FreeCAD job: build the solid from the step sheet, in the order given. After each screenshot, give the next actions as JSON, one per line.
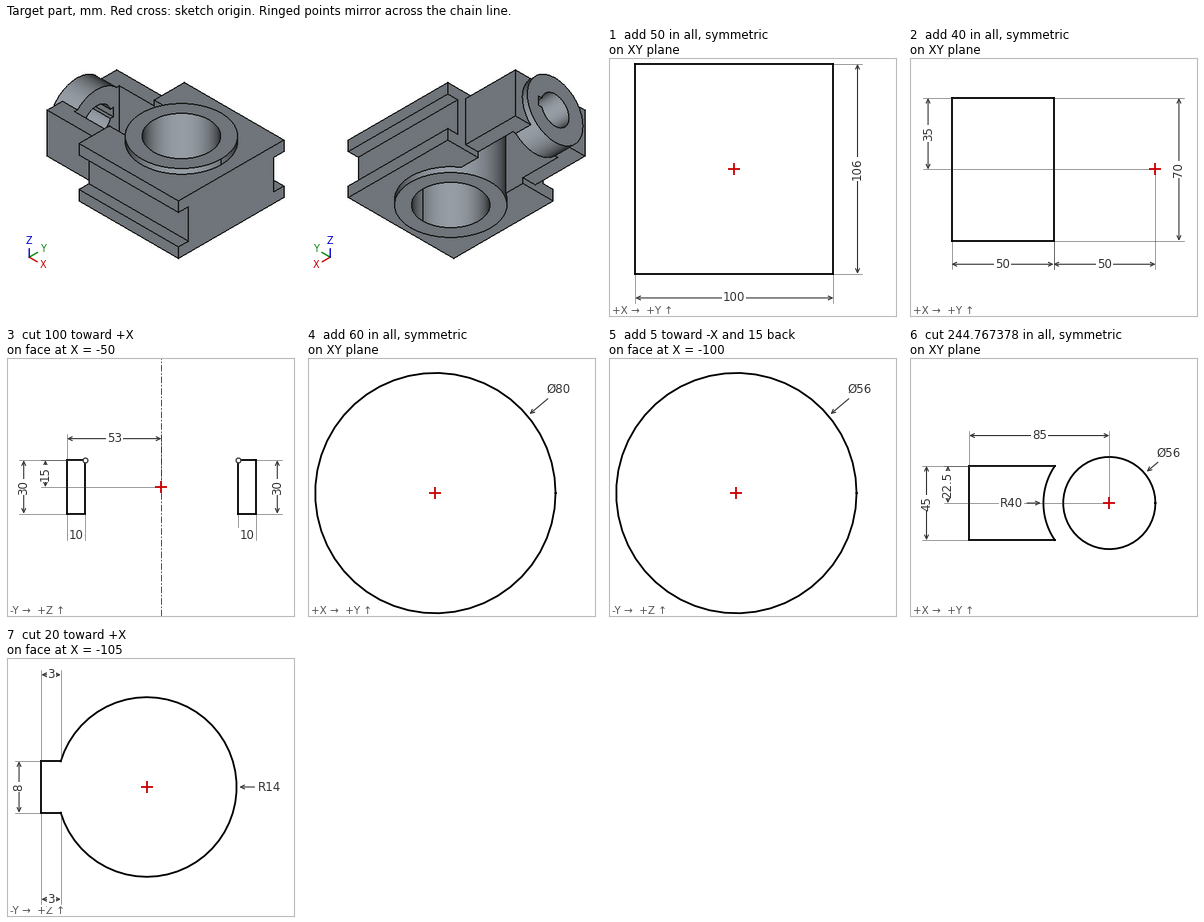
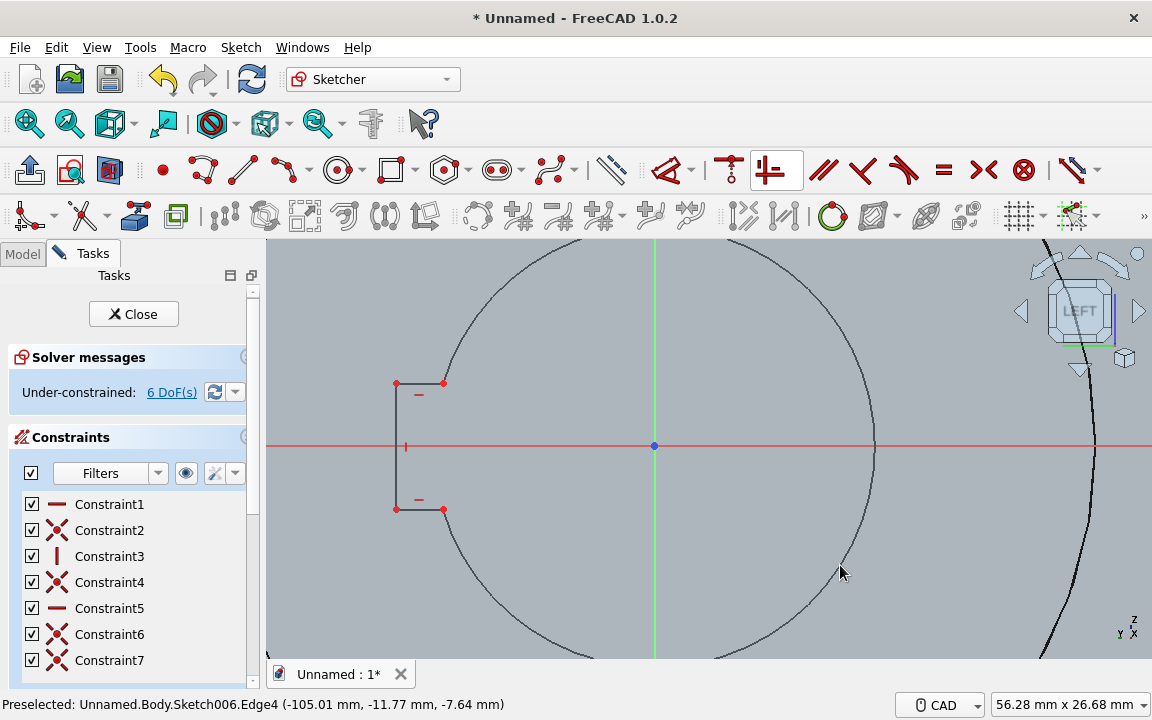
{"action": "left_click_drag", "start_coordinate": [644, 436], "coordinate": [665, 457]}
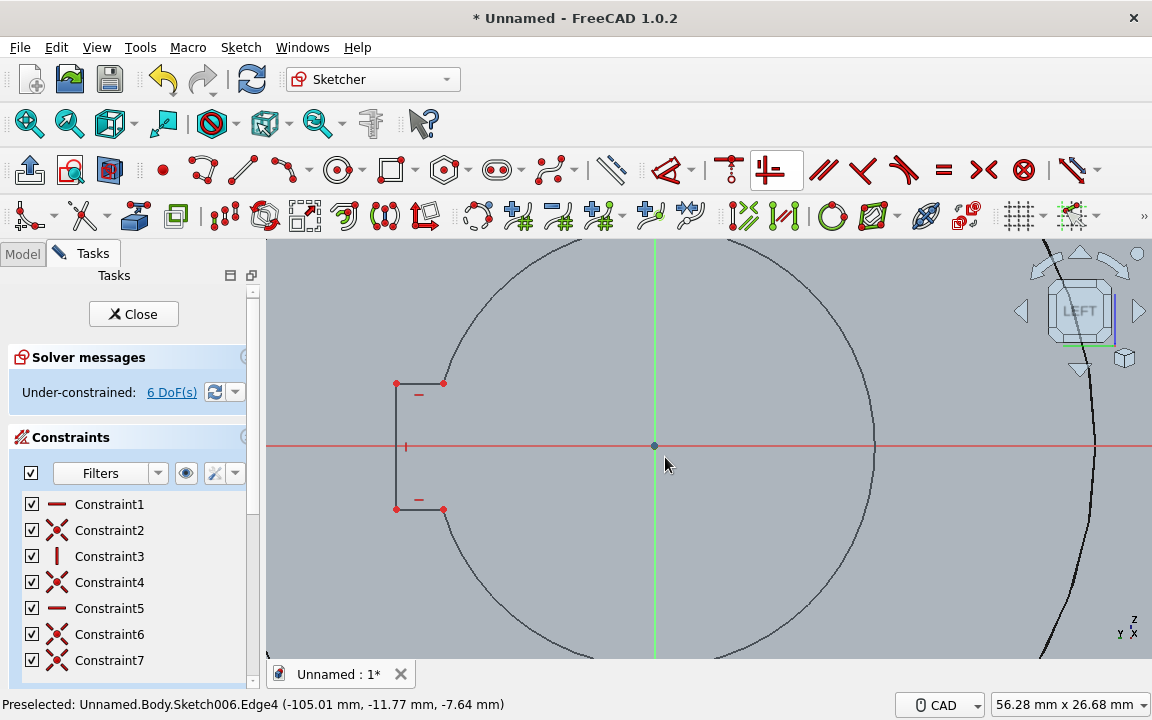
{"action": "left_click", "coordinate": [730, 170]}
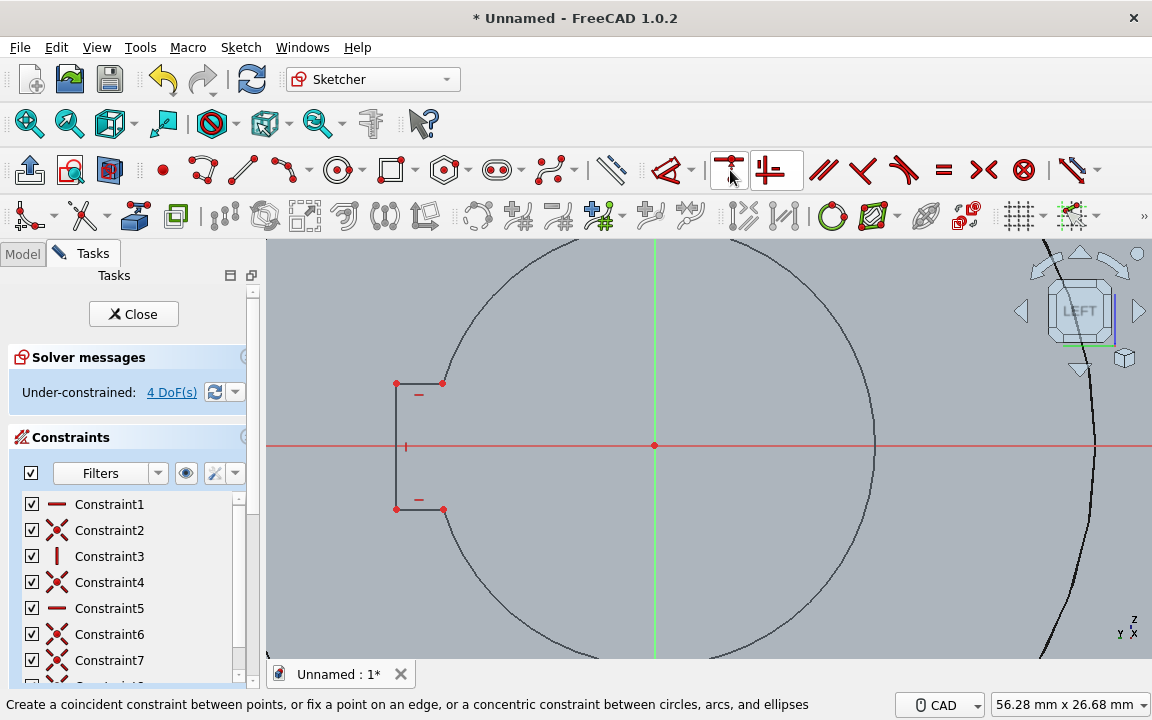
{"action": "left_click", "coordinate": [666, 170]}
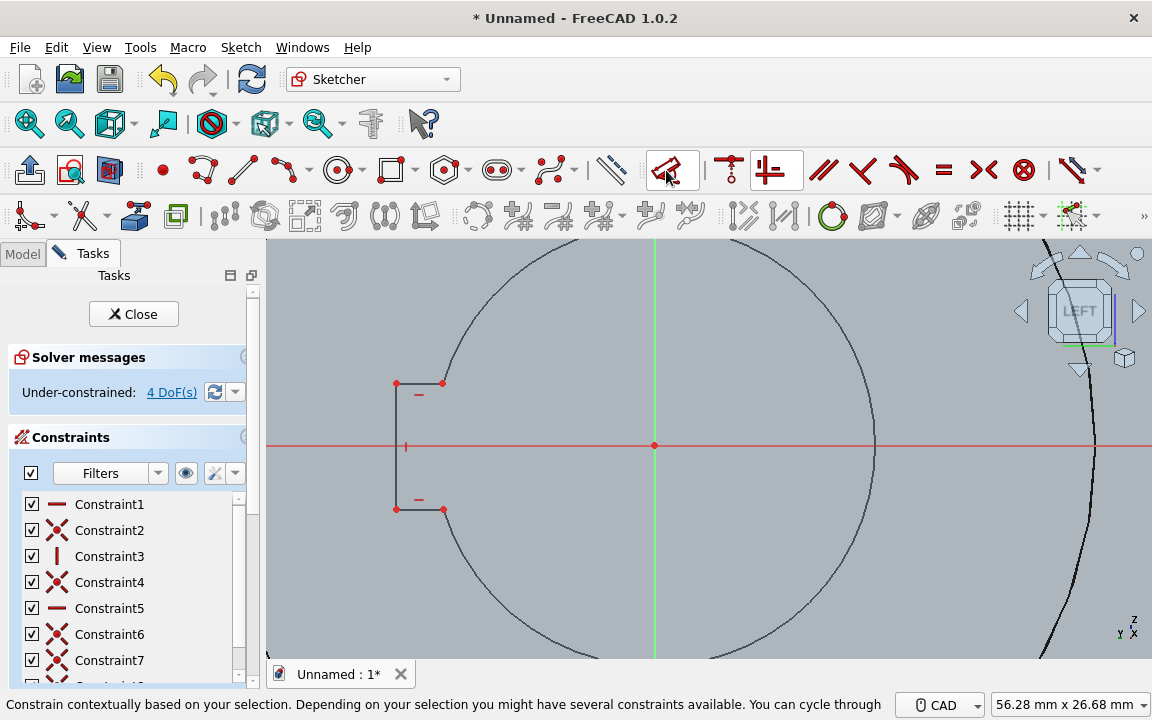
{"action": "left_click", "coordinate": [875, 445]}
{"action": "left_click", "coordinate": [877, 566]}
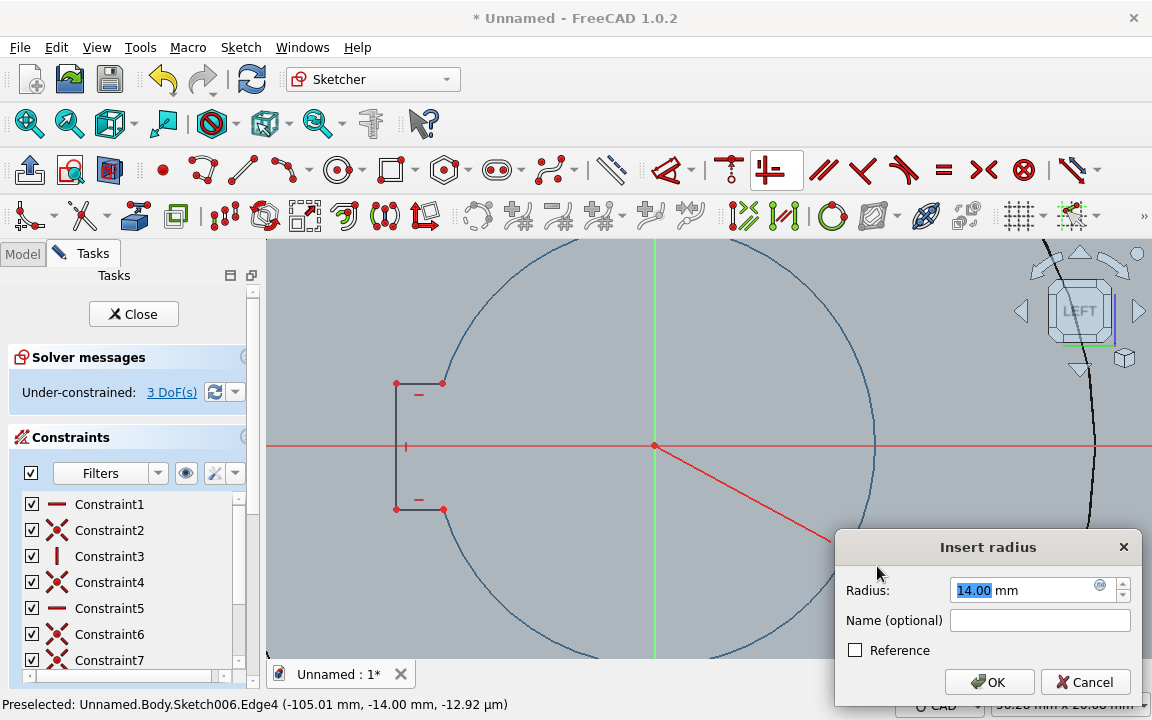
{"action": "type", "text": "14"}
{"action": "key", "text": "Return"}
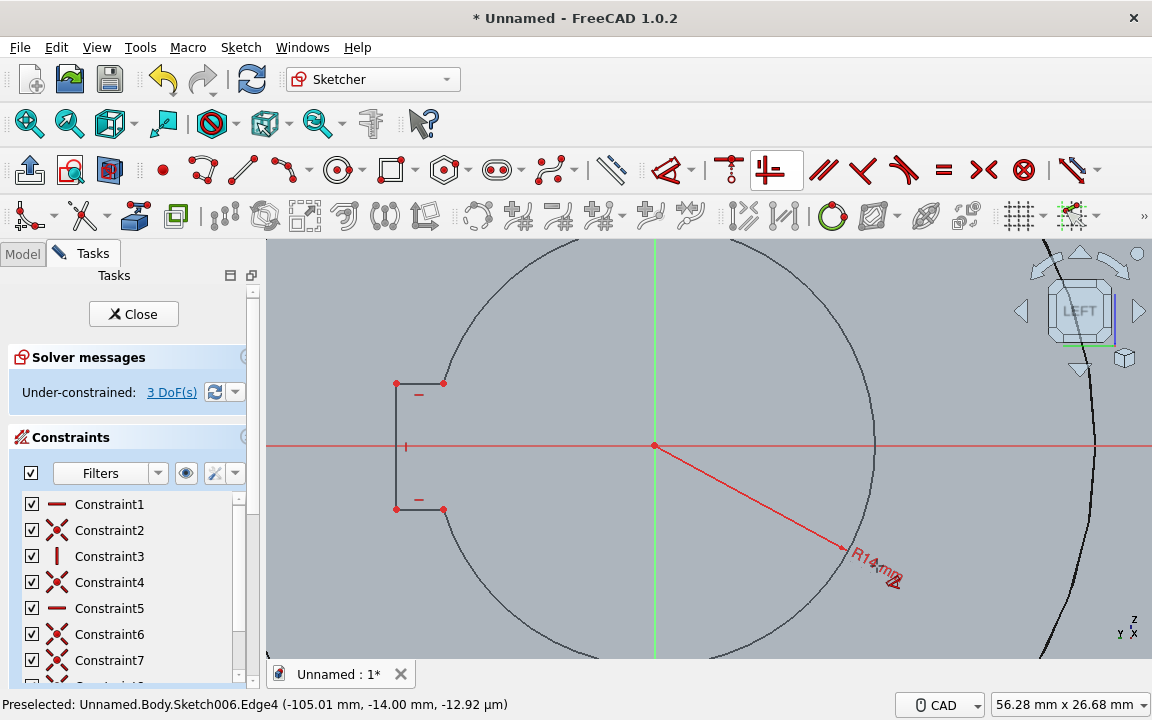
{"action": "left_click", "coordinate": [429, 384]}
{"action": "left_click", "coordinate": [420, 350]}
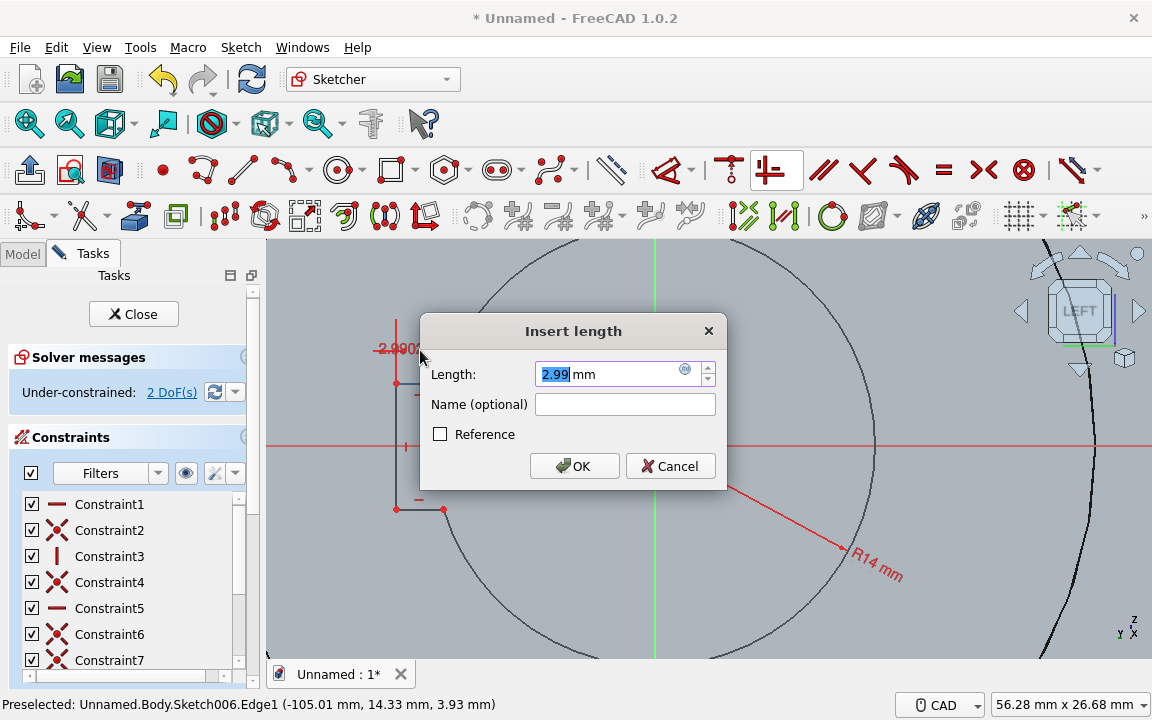
{"action": "type", "text": "3"}
{"action": "key", "text": "Return"}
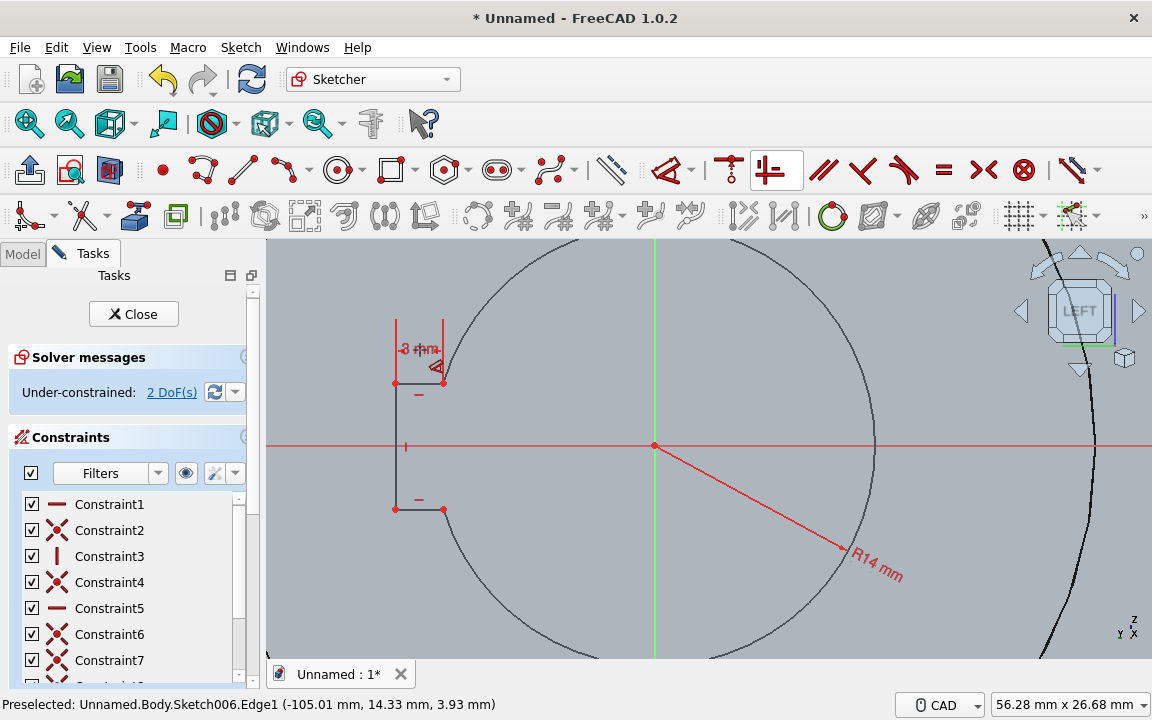
{"action": "left_click", "coordinate": [396, 422]}
{"action": "left_click", "coordinate": [362, 418]}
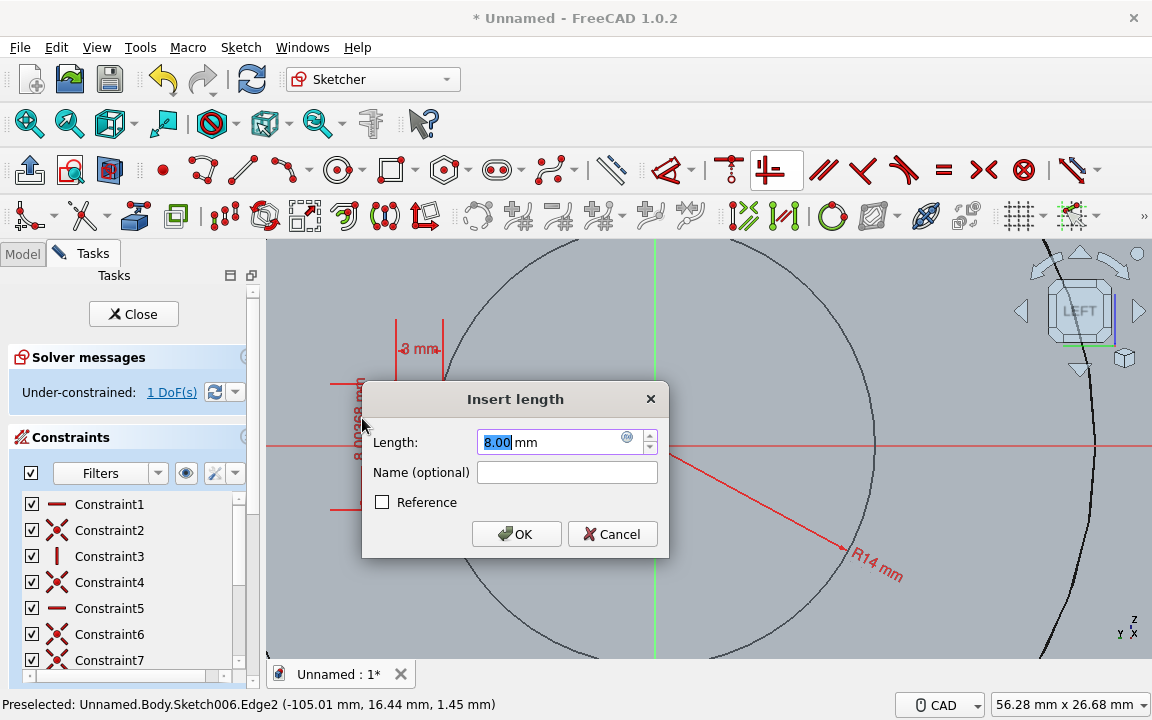
{"action": "type", "text": "8"}
{"action": "key", "text": "Return"}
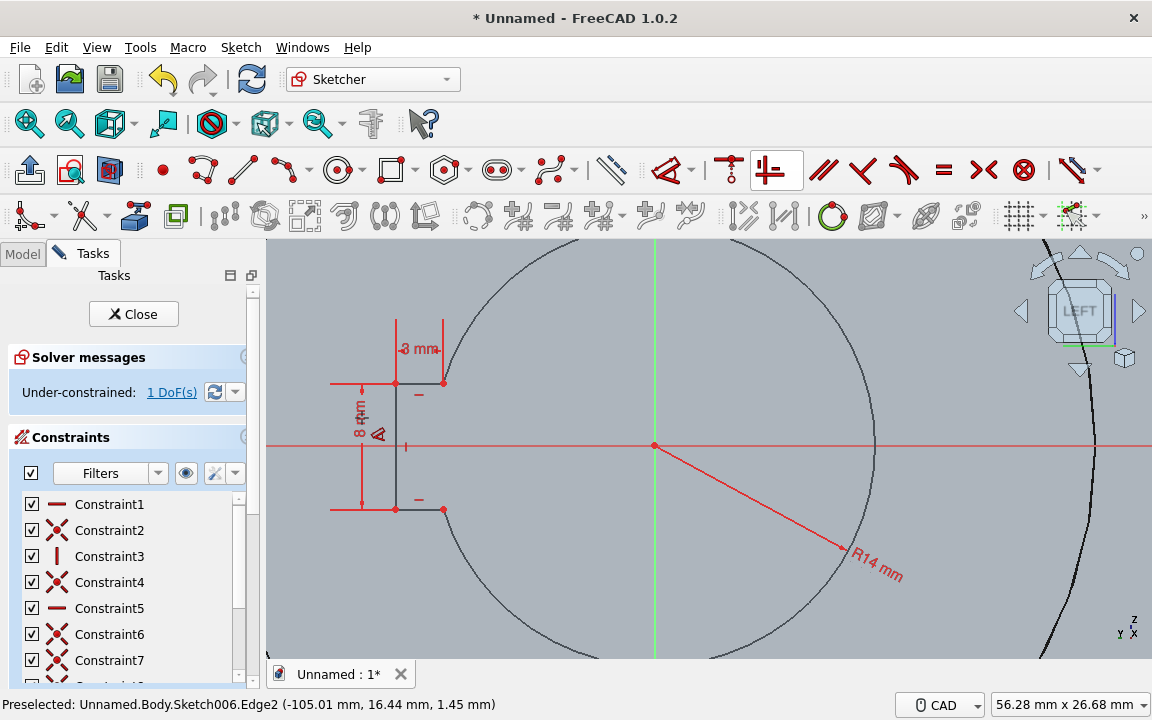
{"action": "left_click", "coordinate": [410, 510]}
{"action": "left_click", "coordinate": [420, 544]}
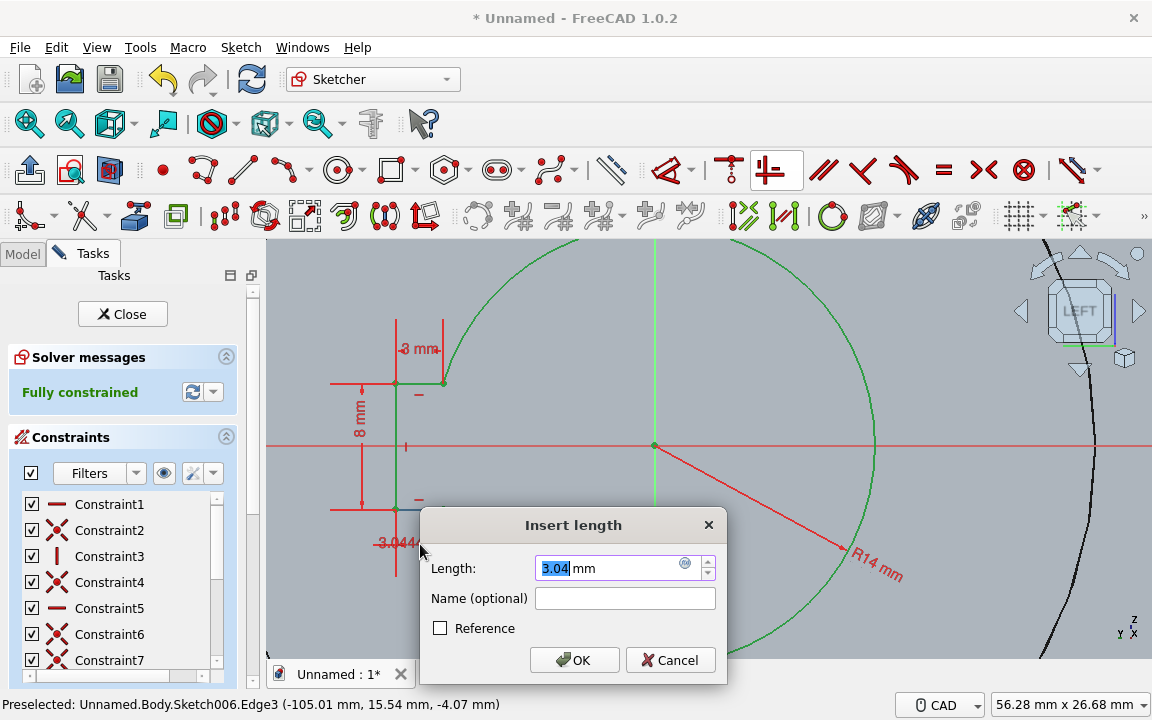
{"action": "type", "text": "3"}
{"action": "key", "text": "Return"}
{"action": "key", "text": "Escape"}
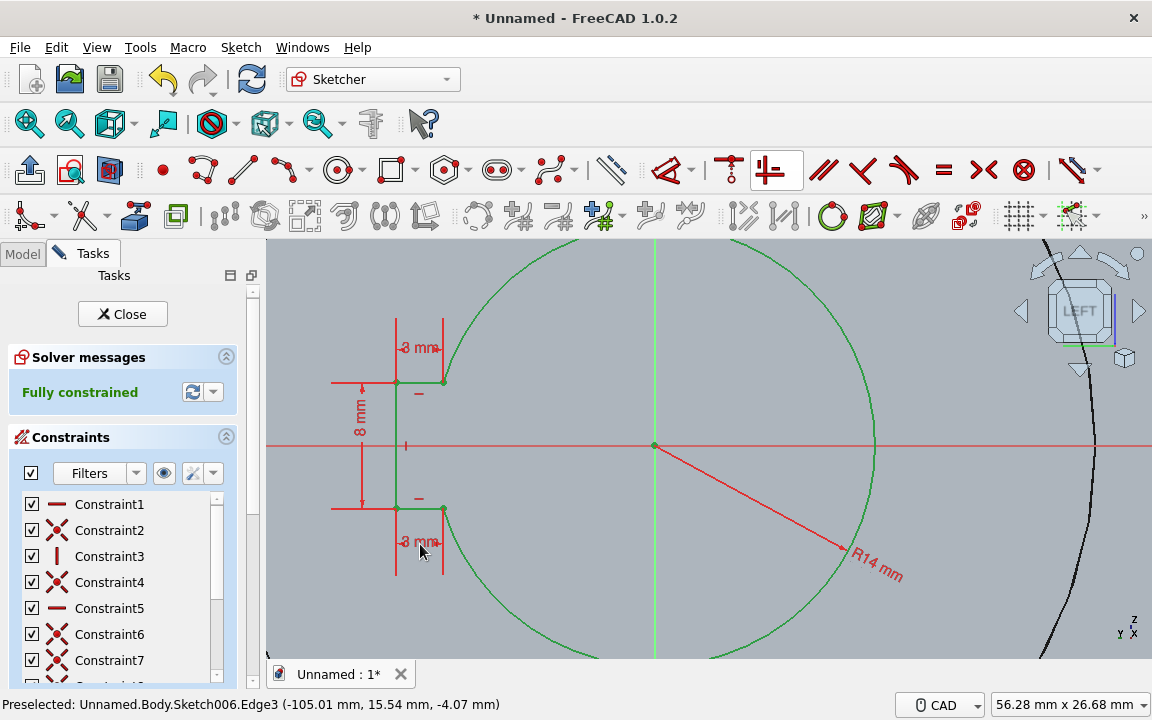
{"action": "left_click", "coordinate": [123, 314]}